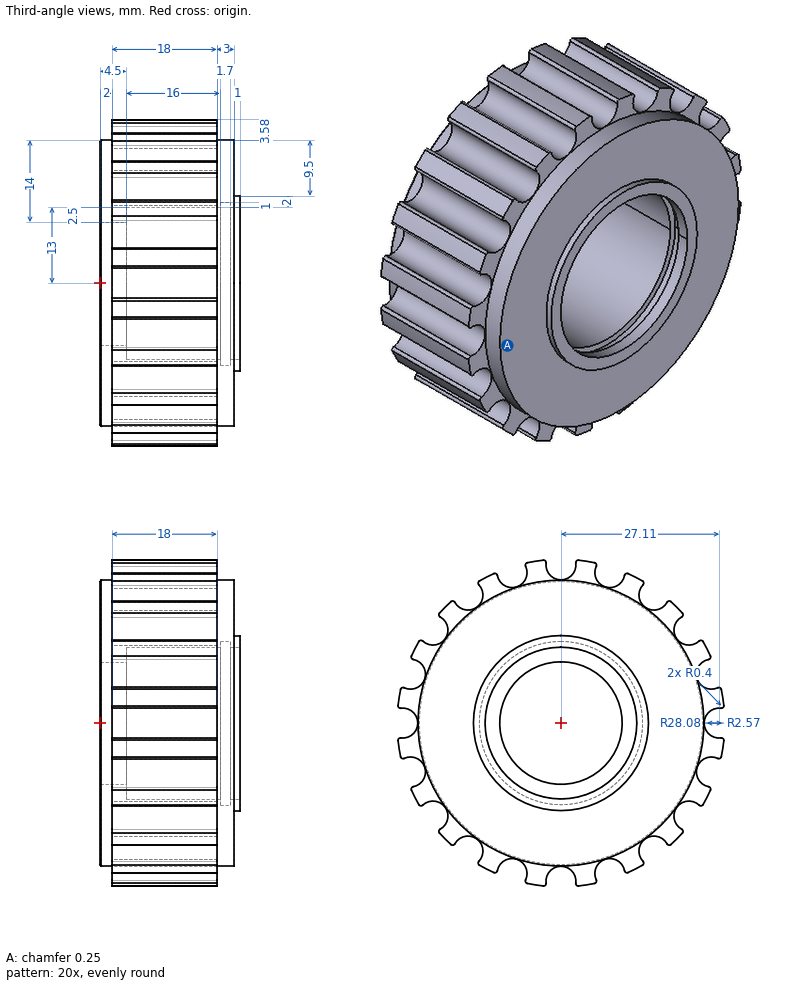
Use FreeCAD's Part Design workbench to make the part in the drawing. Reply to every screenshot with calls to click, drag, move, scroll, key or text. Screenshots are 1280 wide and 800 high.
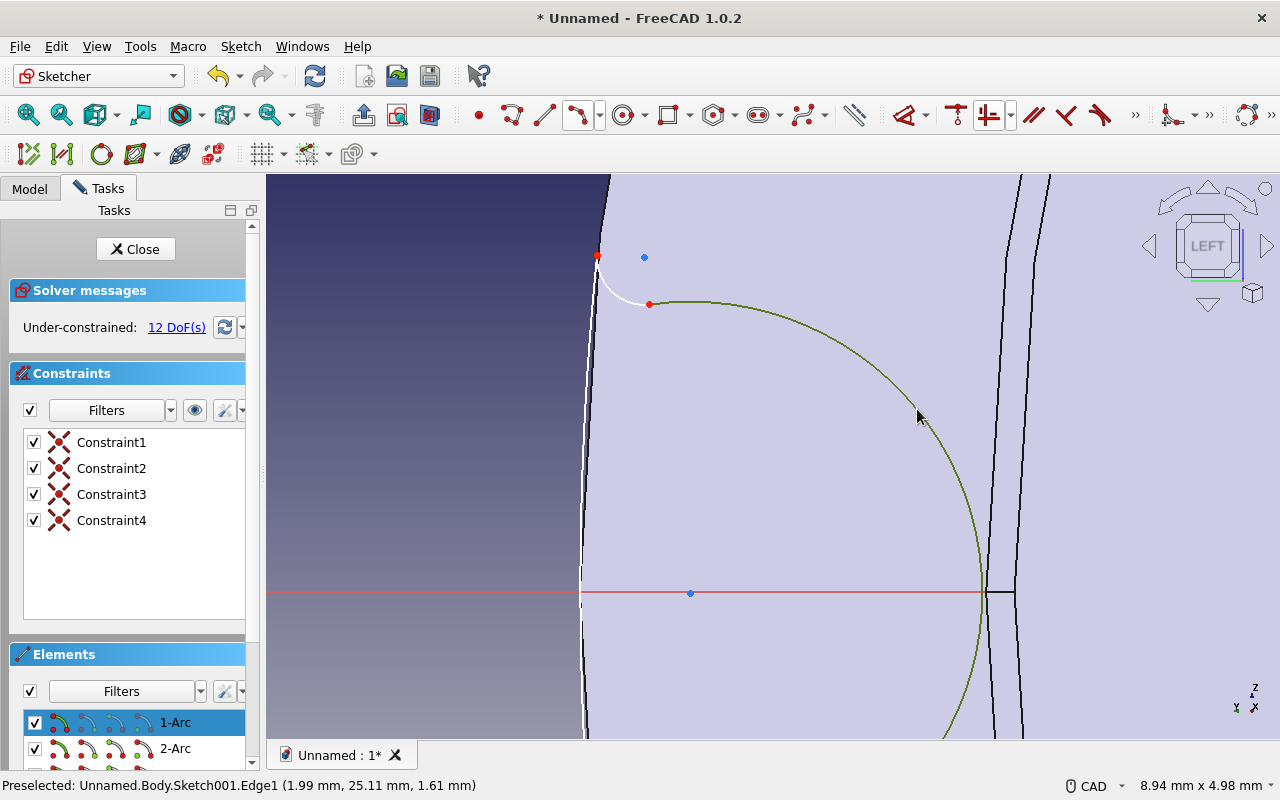
scroll(612, 291, down, 3)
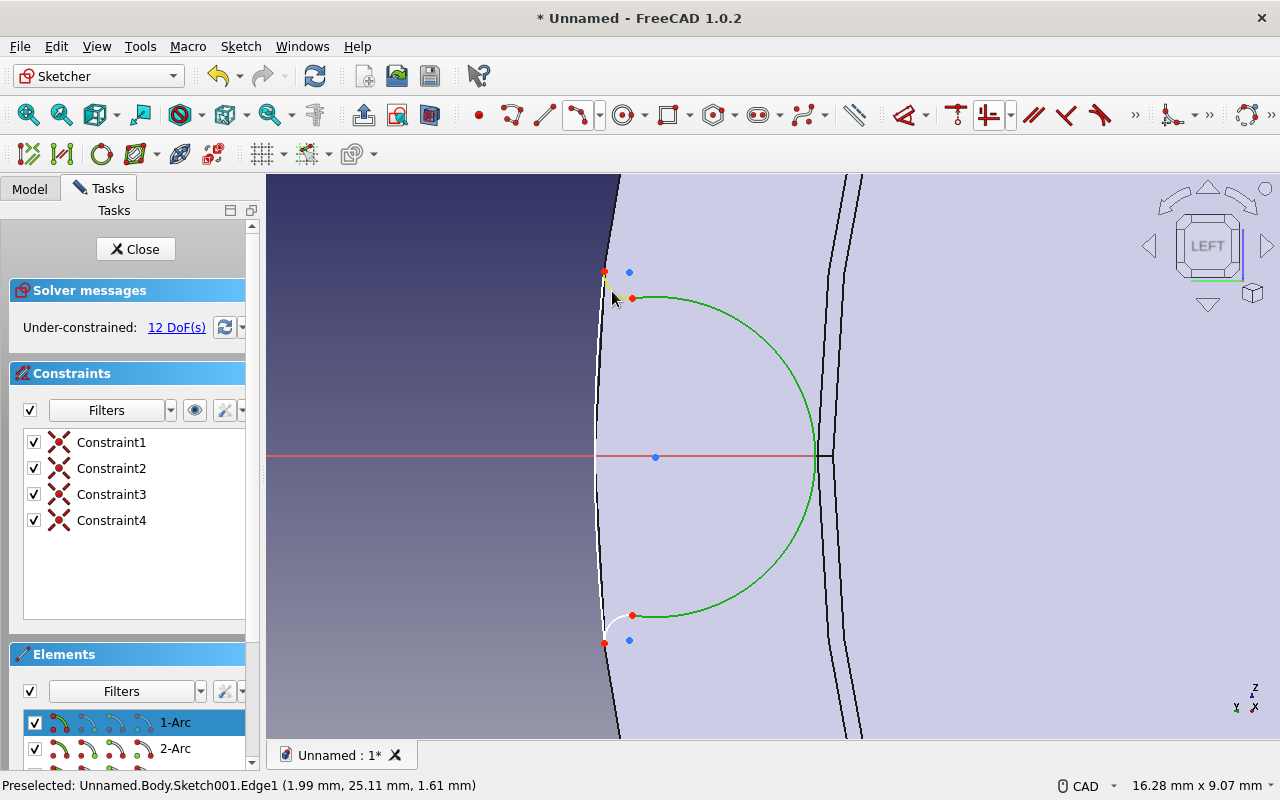
click(619, 617)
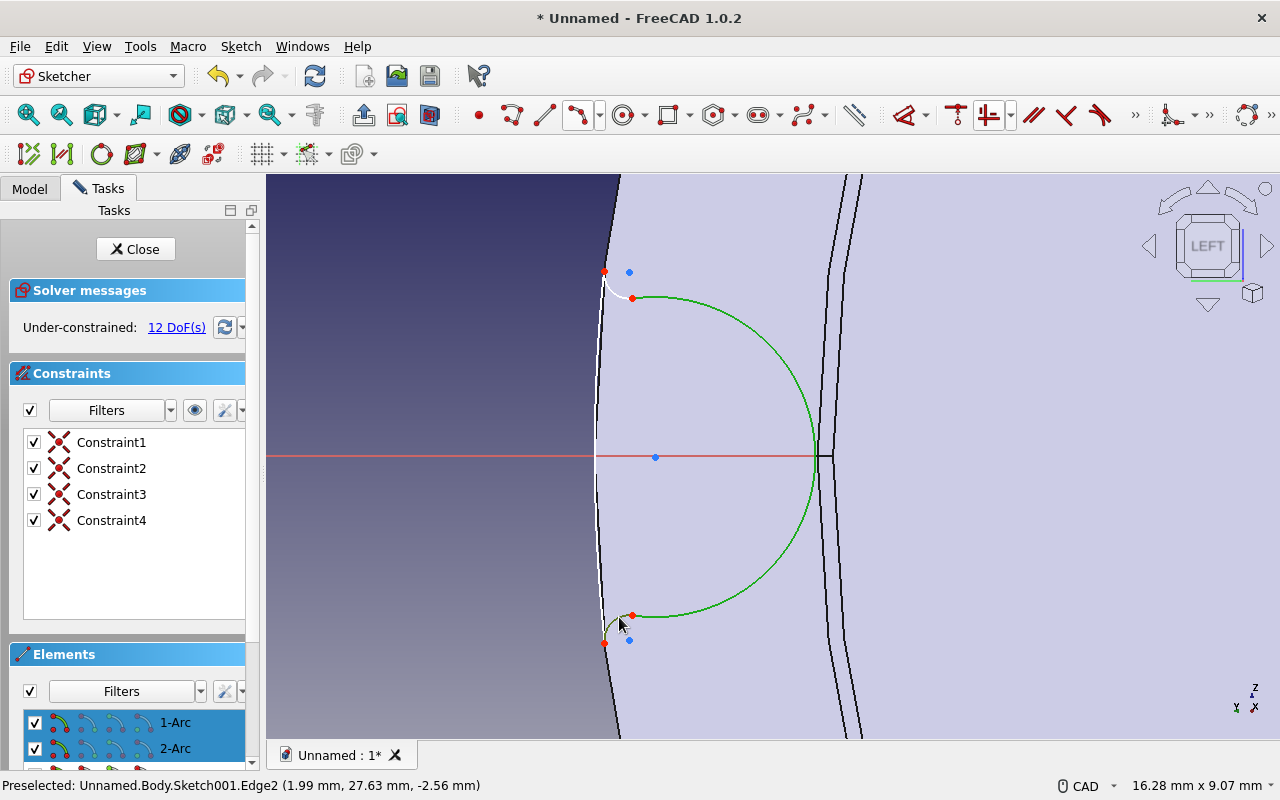
click(1100, 116)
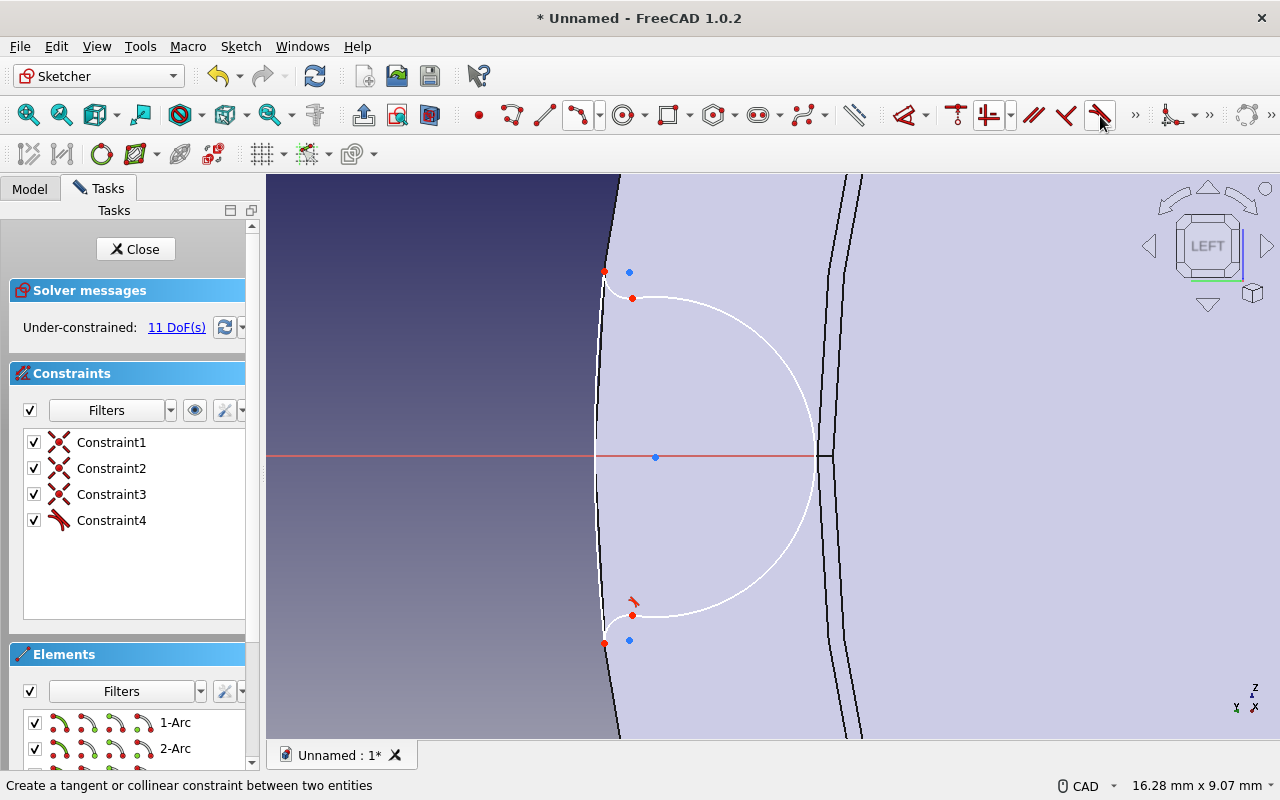
click(779, 558)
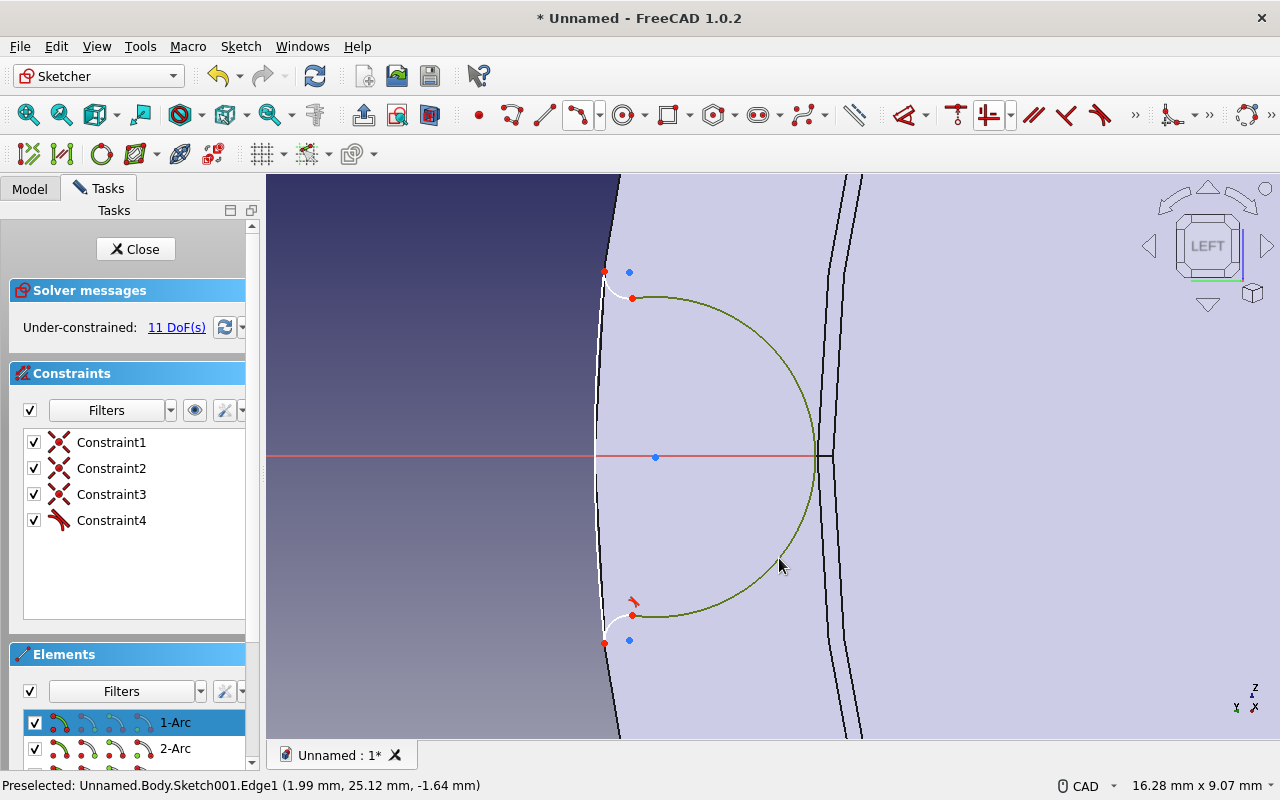
click(620, 297)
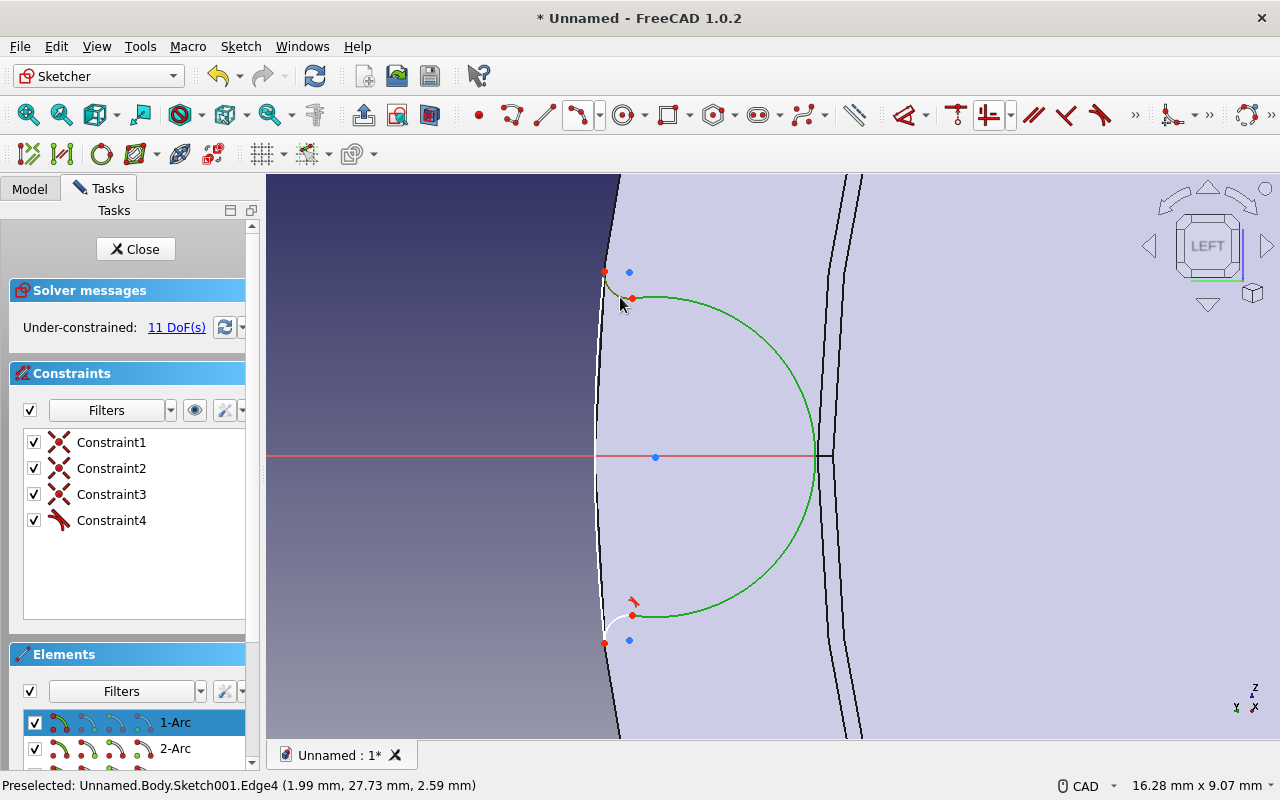
click(1100, 116)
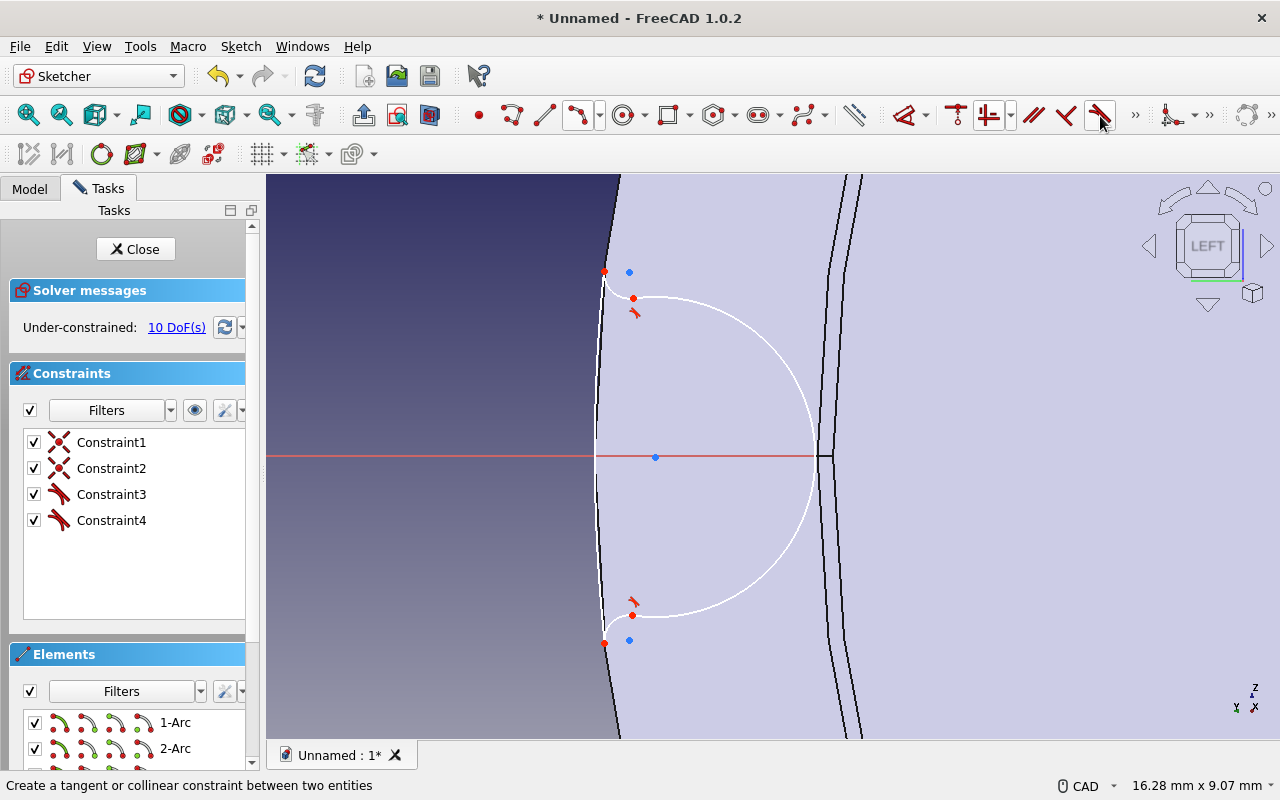
click(619, 617)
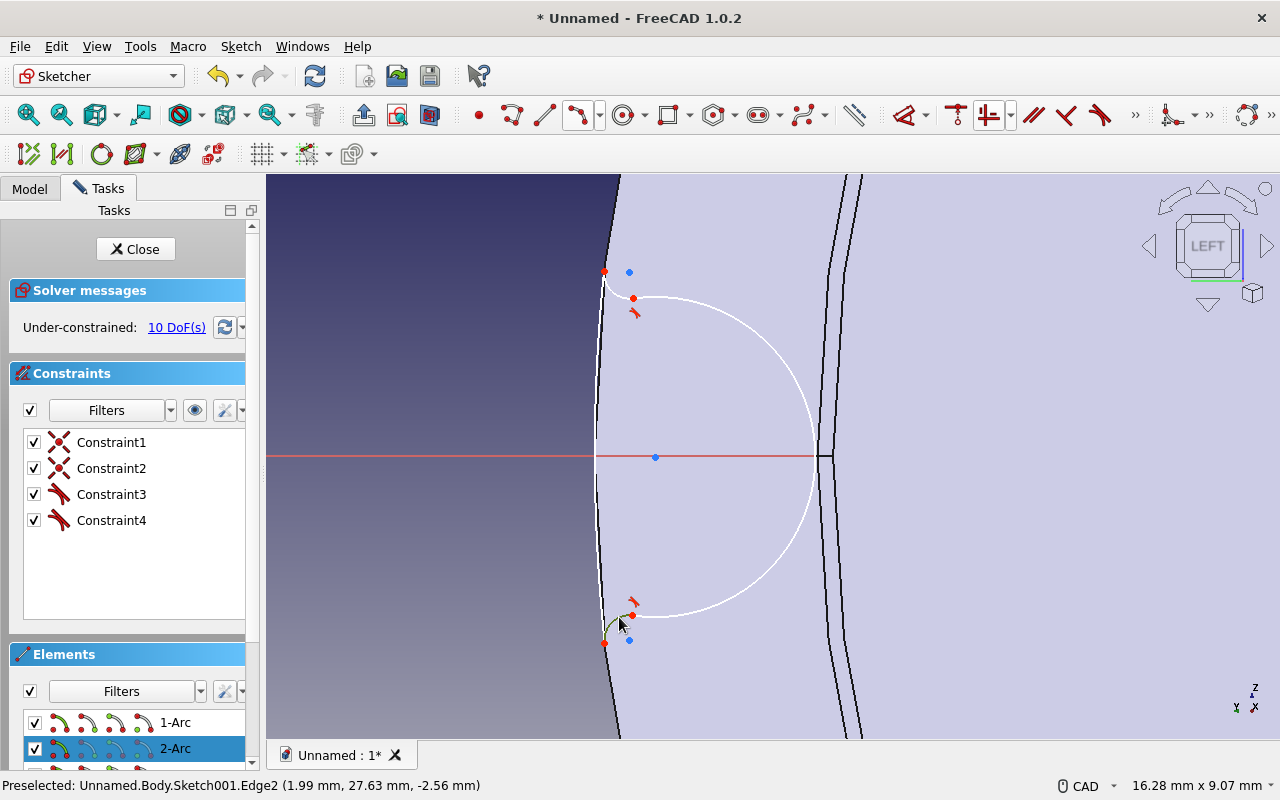
click(596, 383)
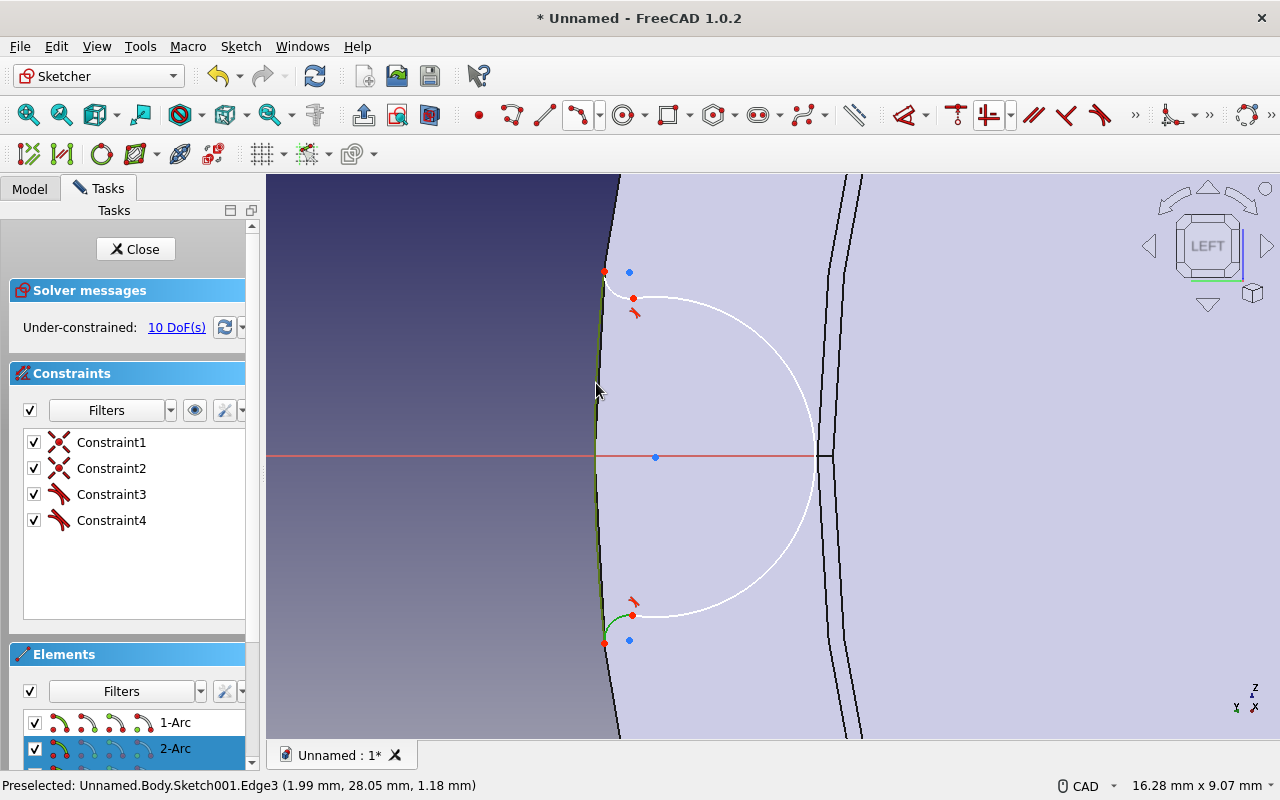
click(1100, 116)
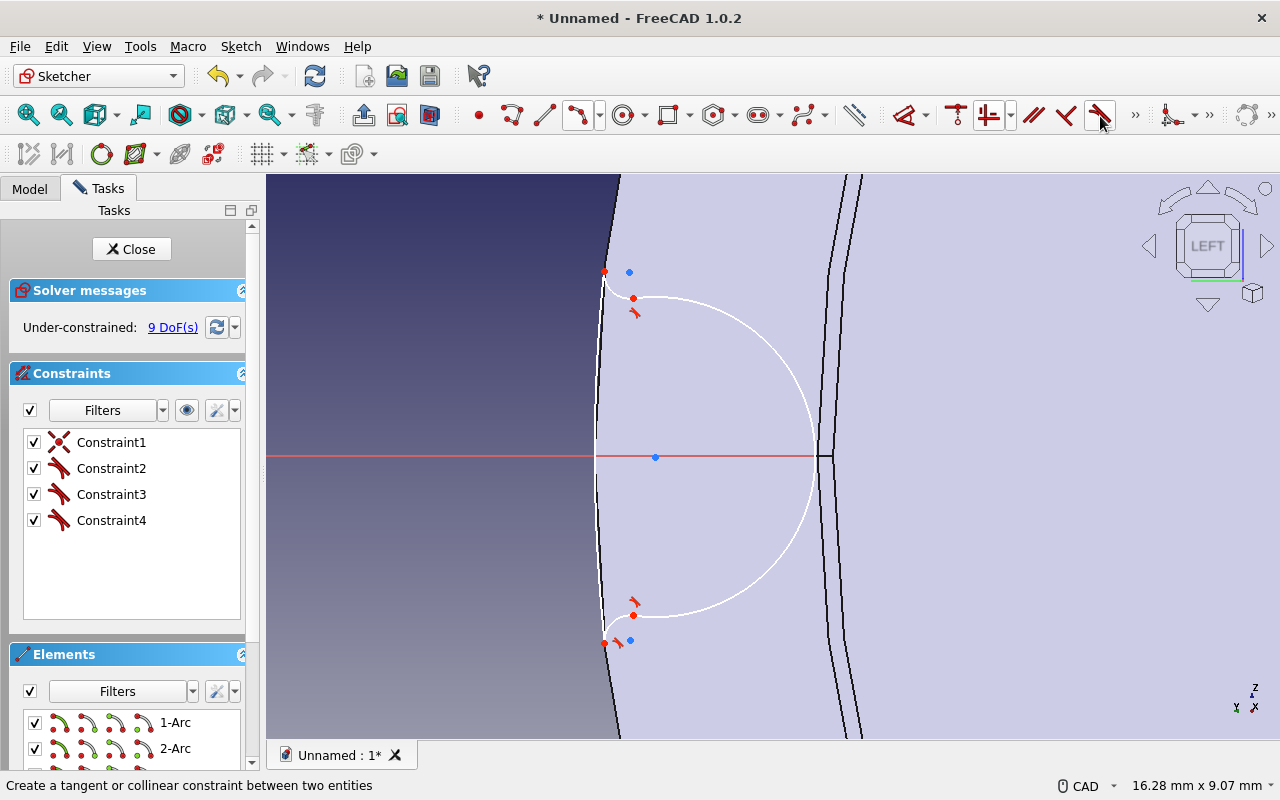
click(596, 383)